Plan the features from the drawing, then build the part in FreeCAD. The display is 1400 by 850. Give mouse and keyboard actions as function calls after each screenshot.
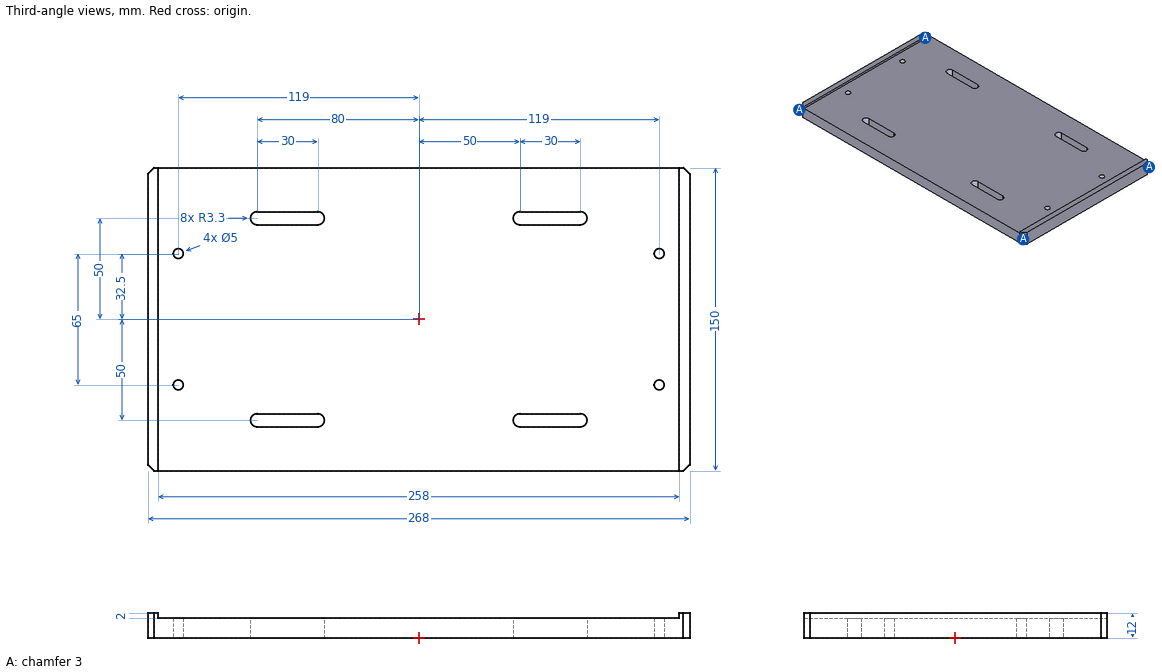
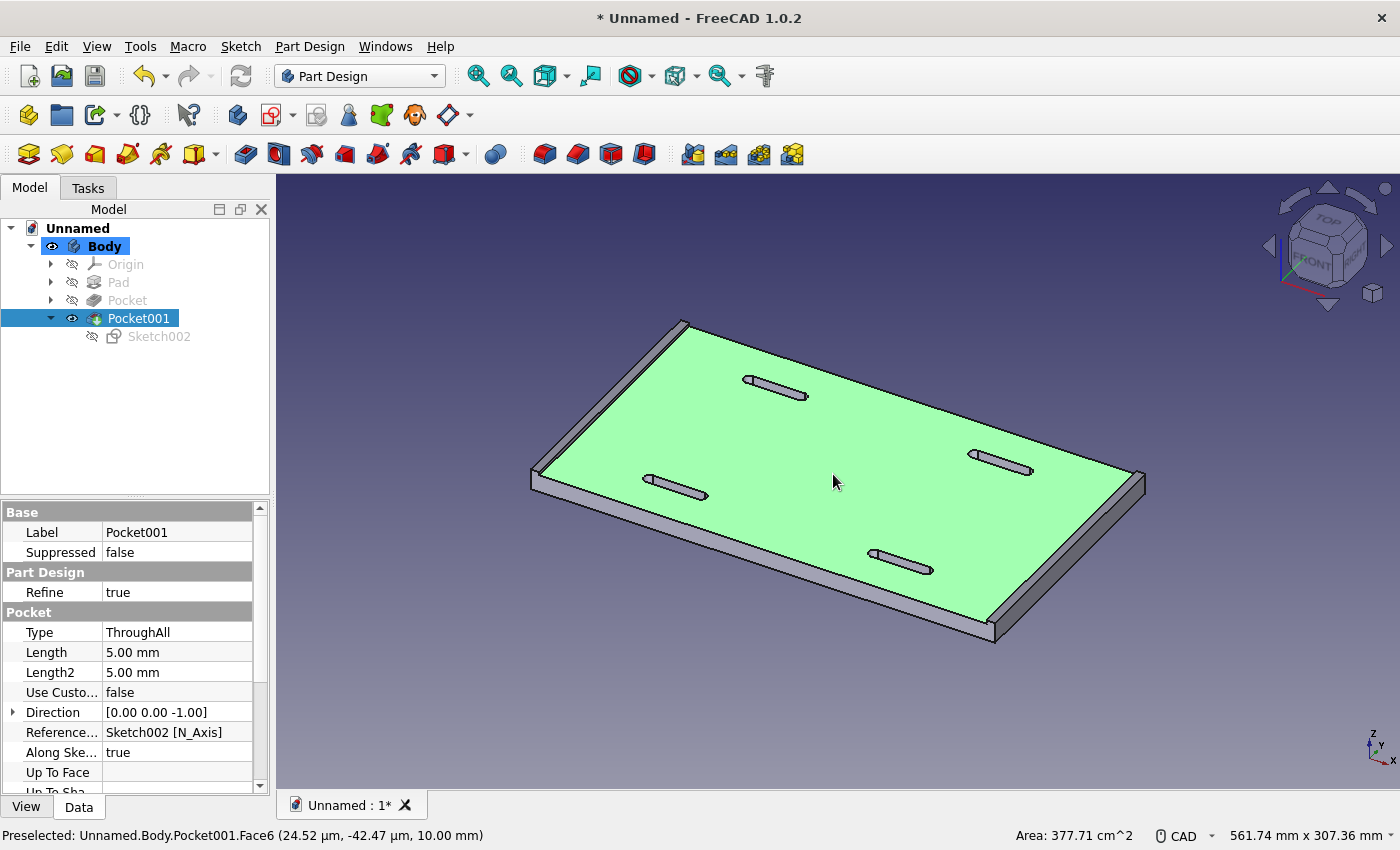
click(270, 116)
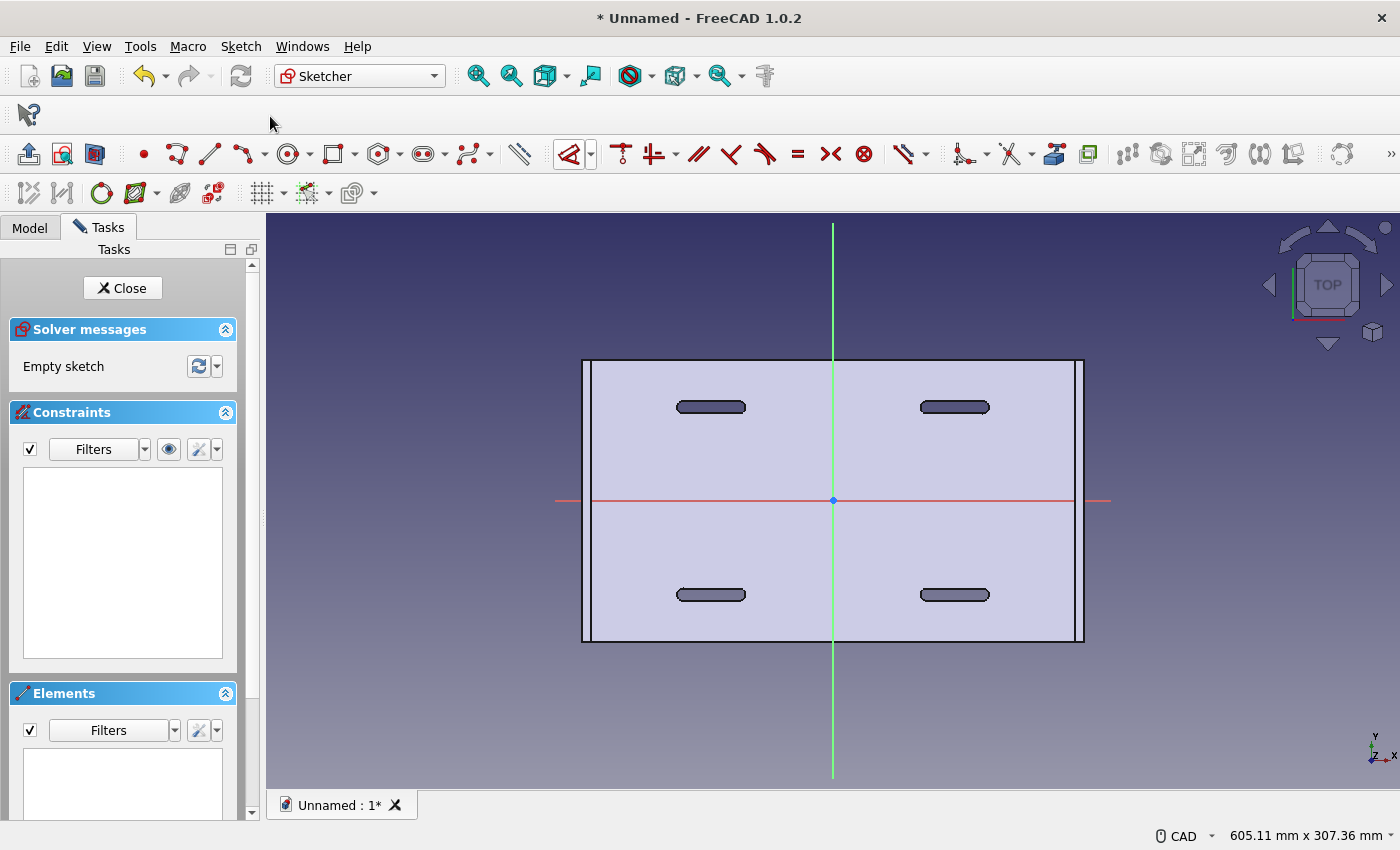
click(95, 154)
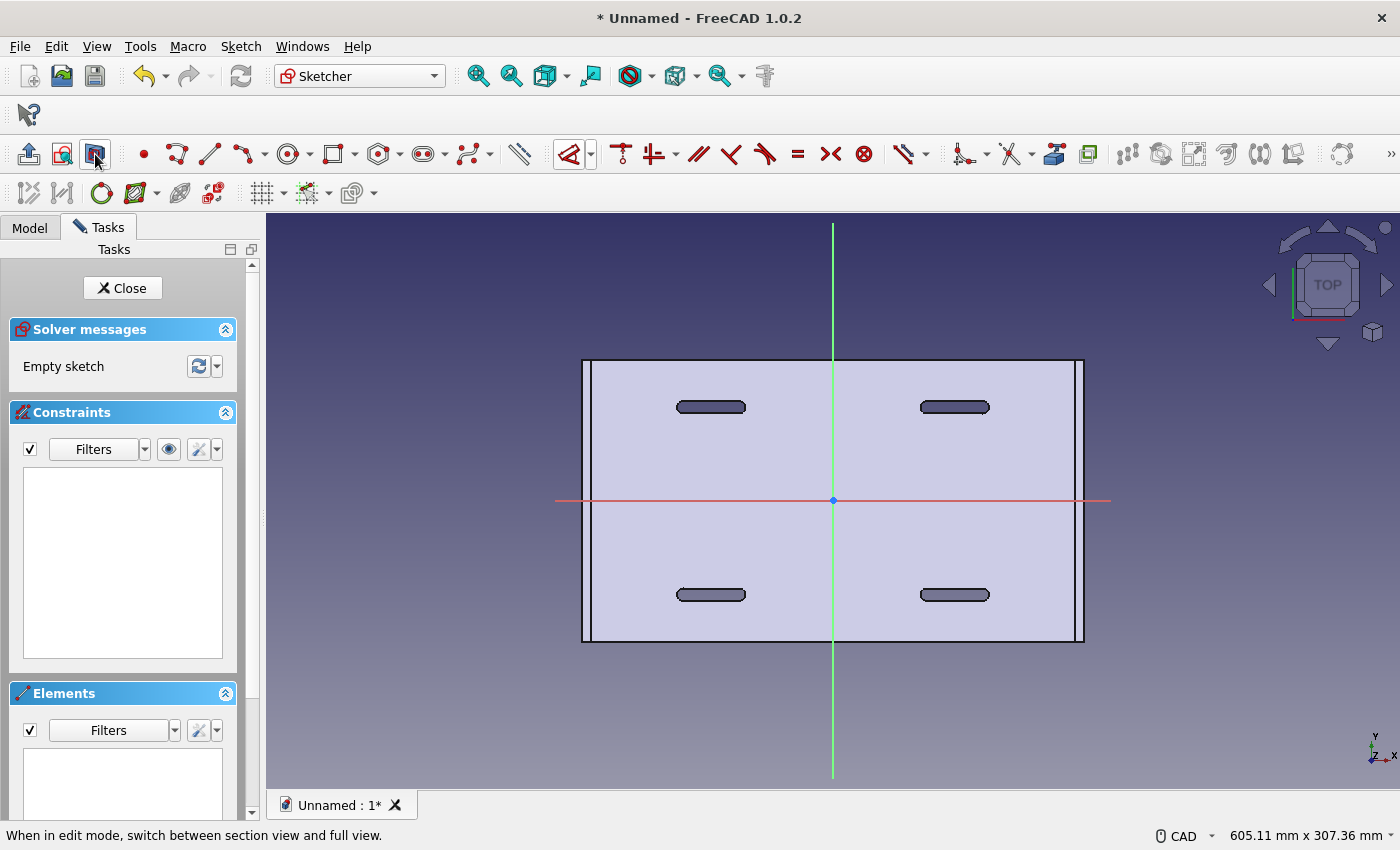
scroll(972, 501, up, 2)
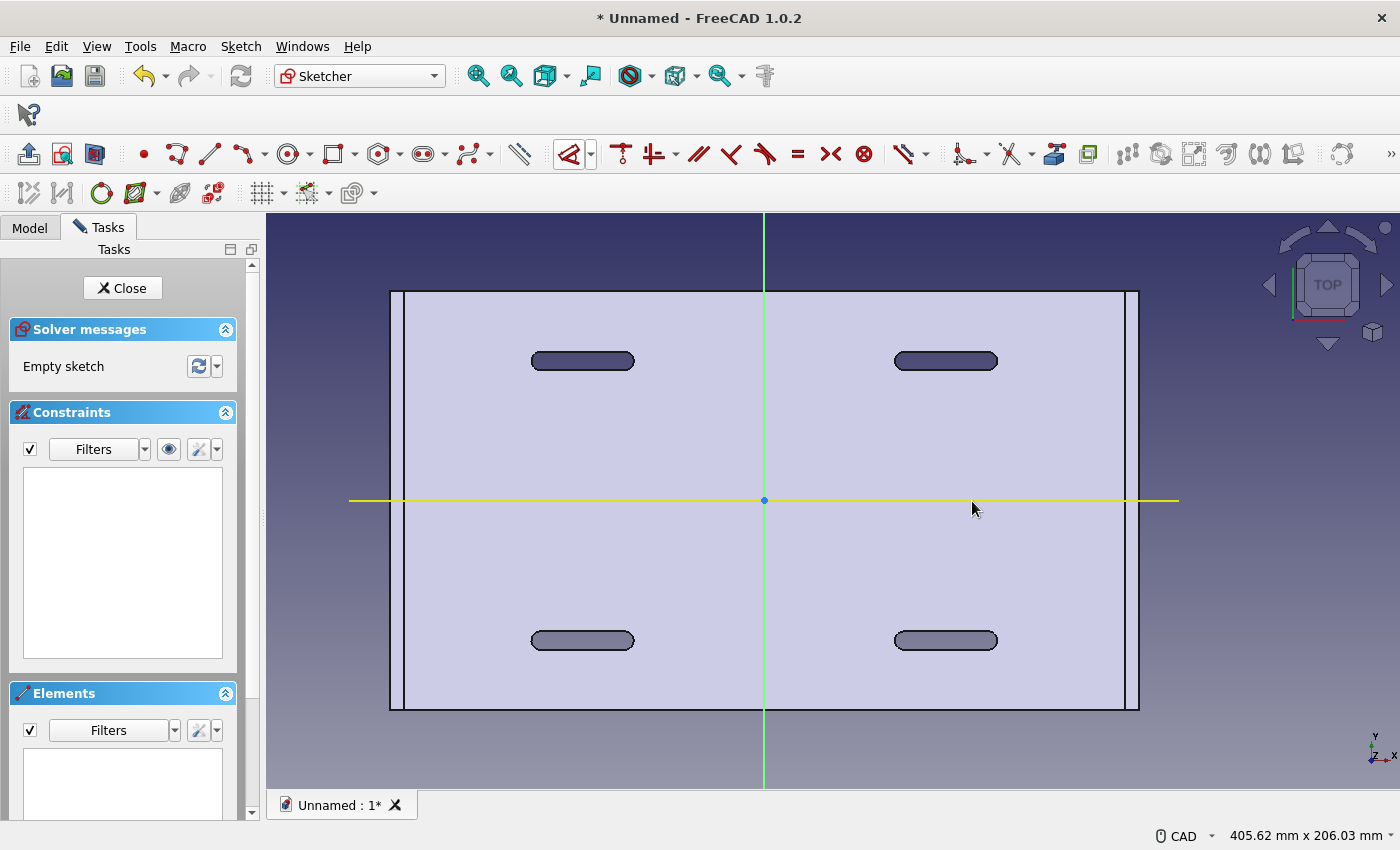
click(288, 154)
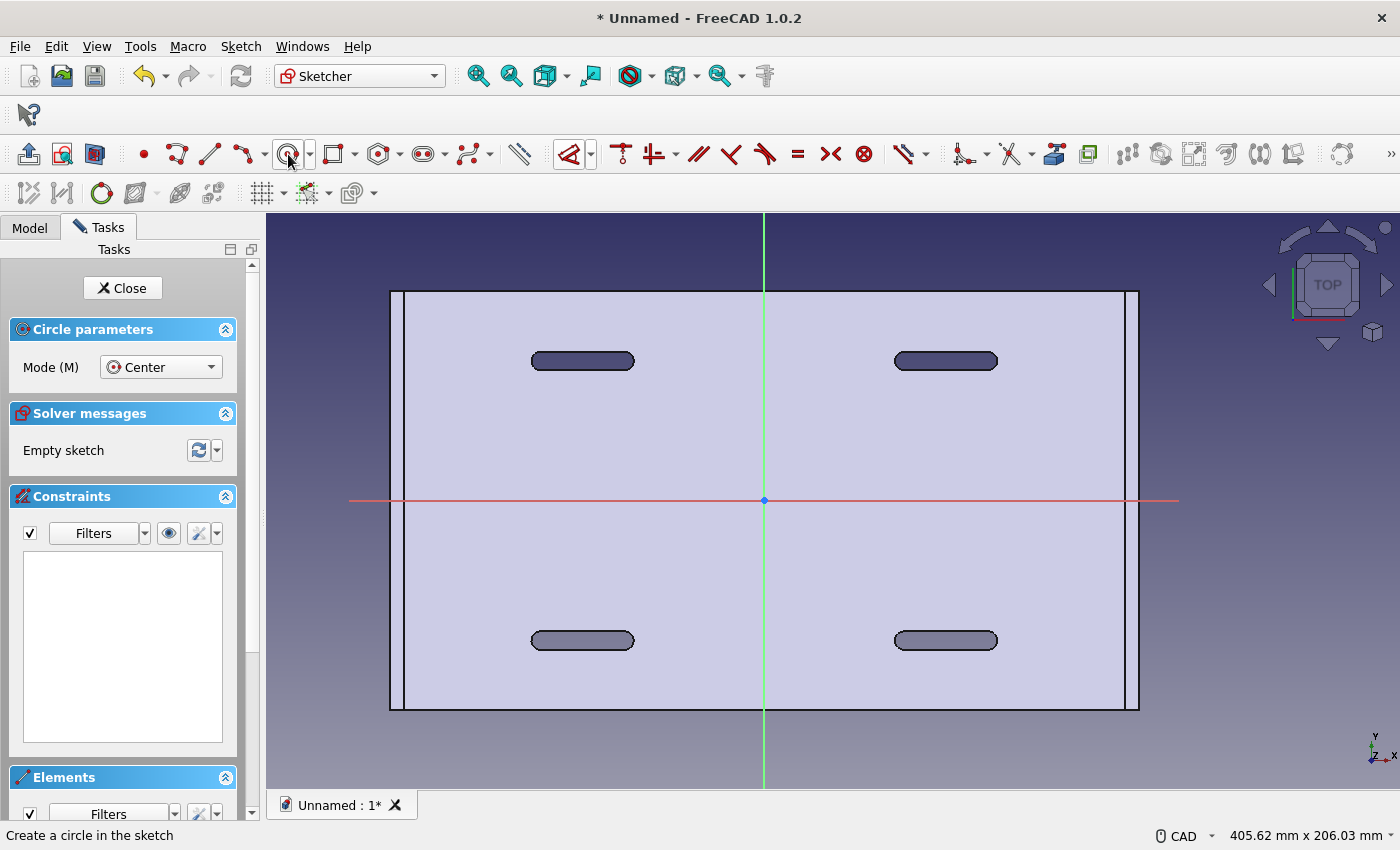
scroll(432, 410, up, 6)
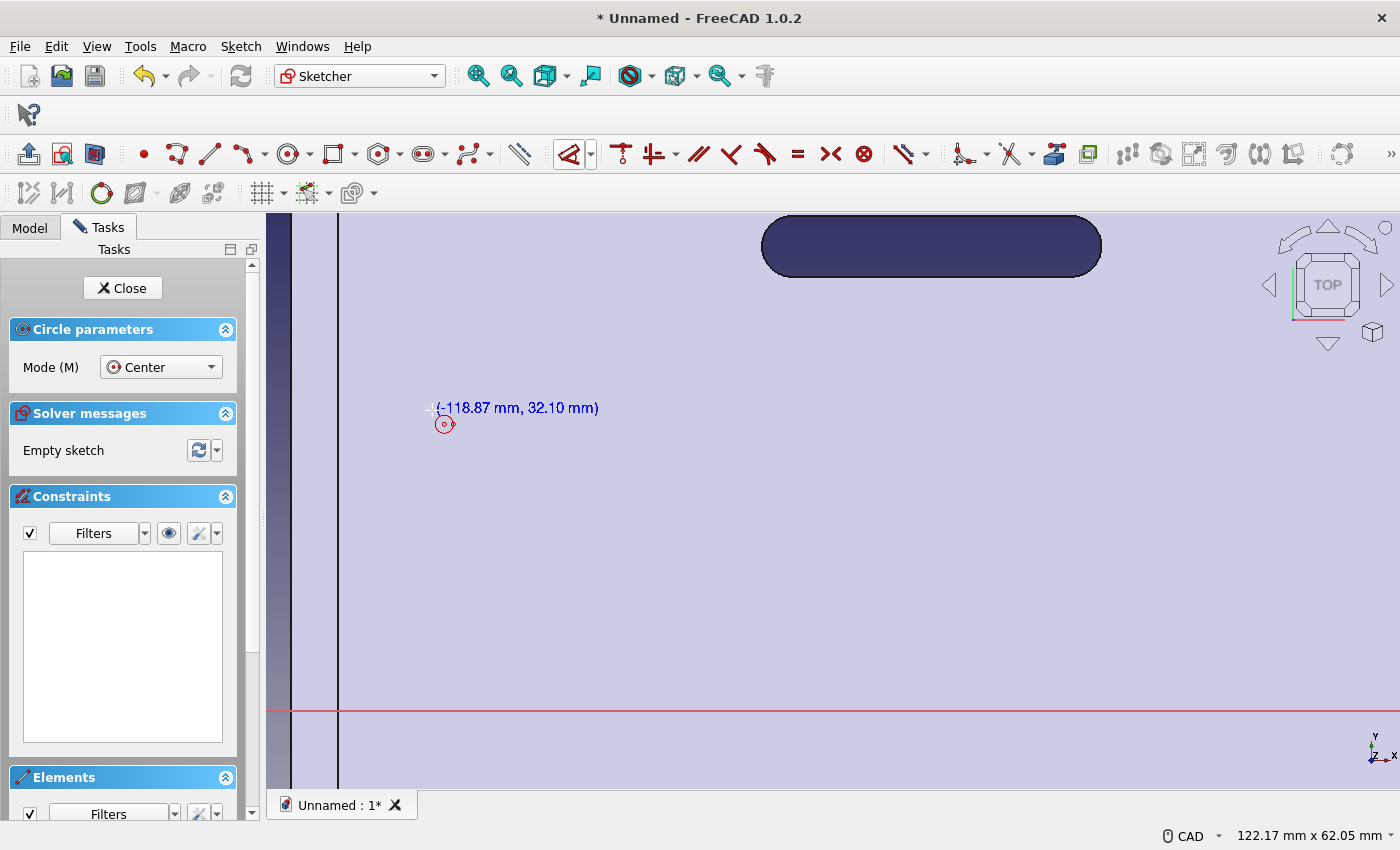
click(430, 409)
move(447, 392)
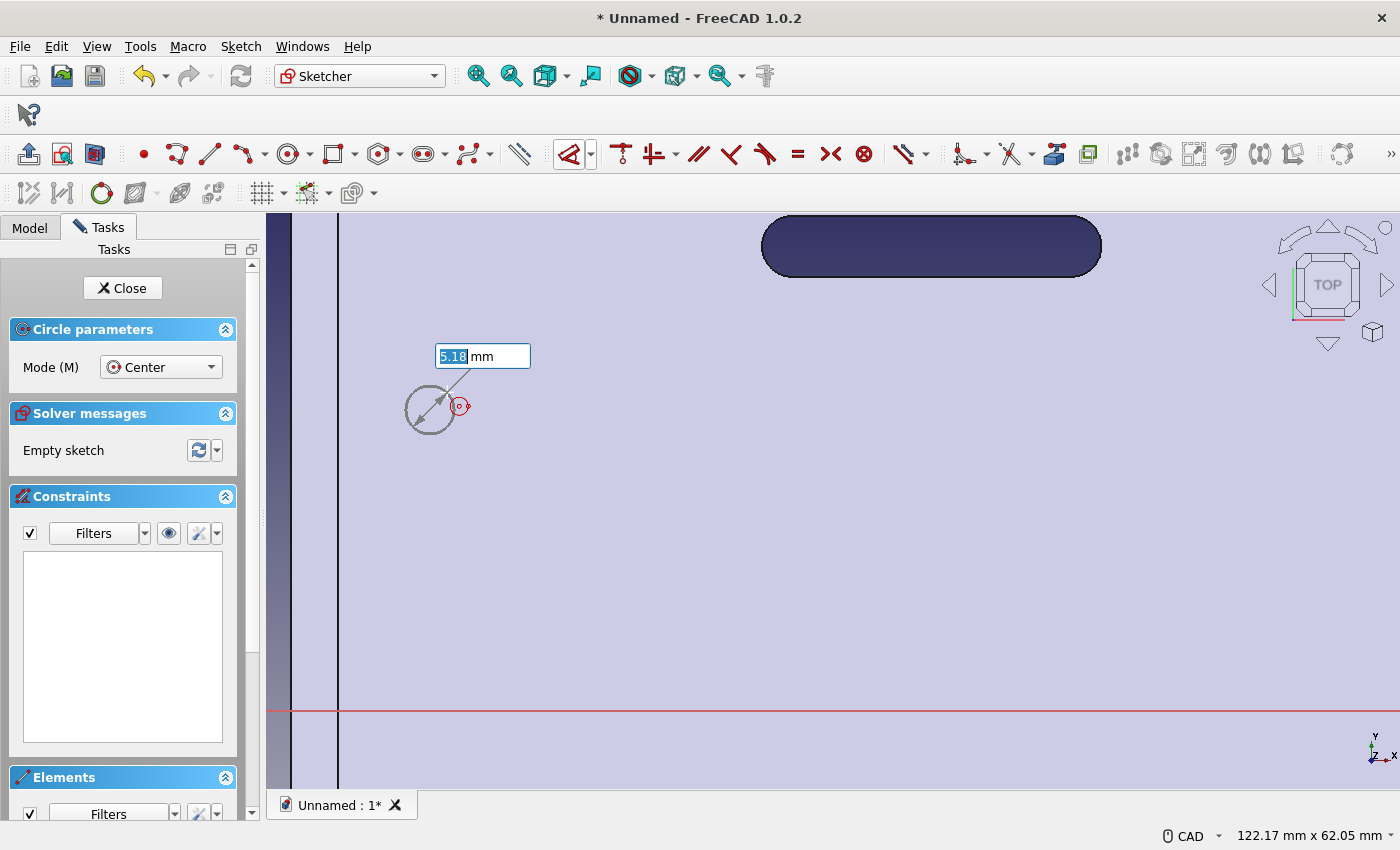
text(5)
key(Return)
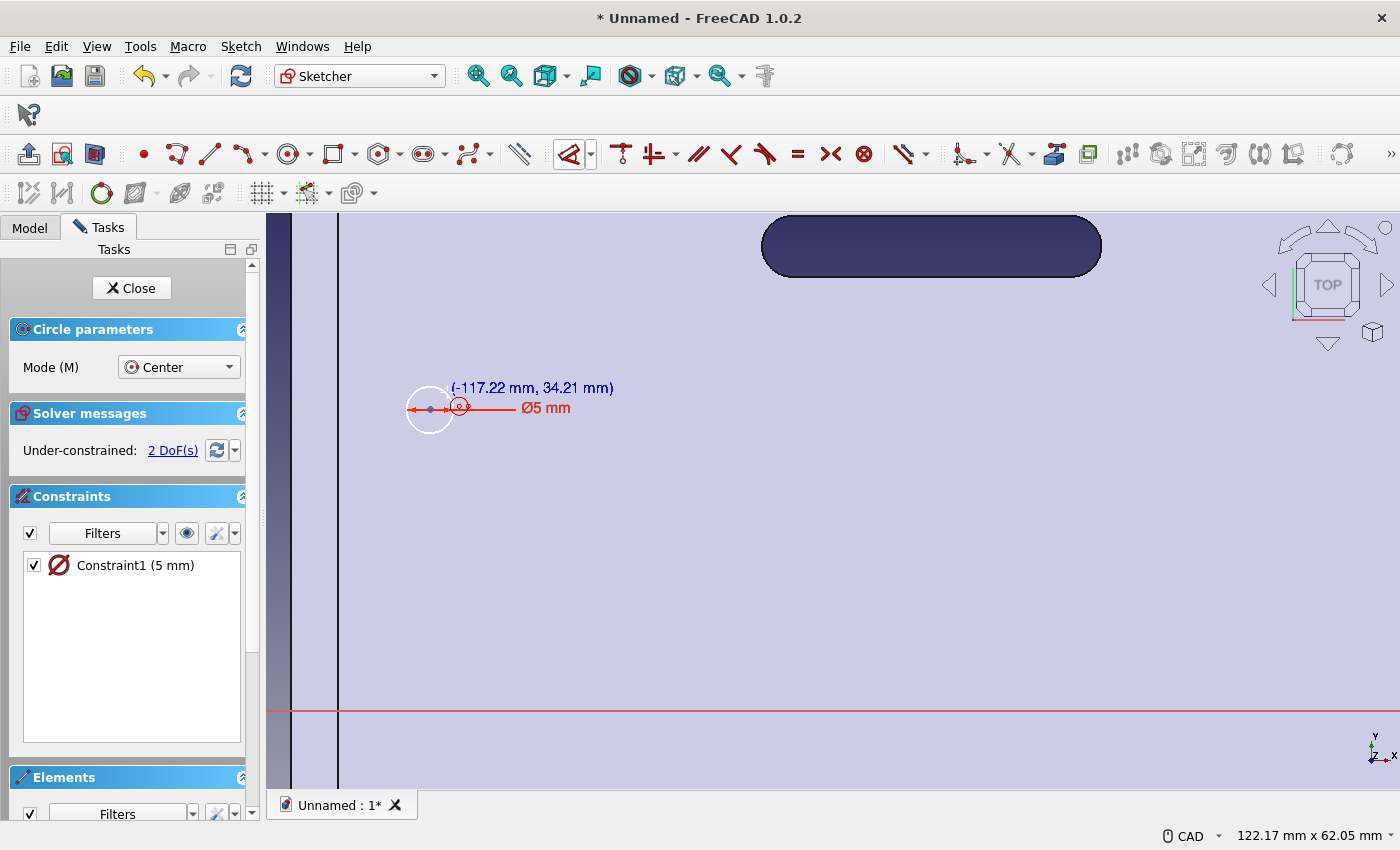
scroll(432, 411, down, 6)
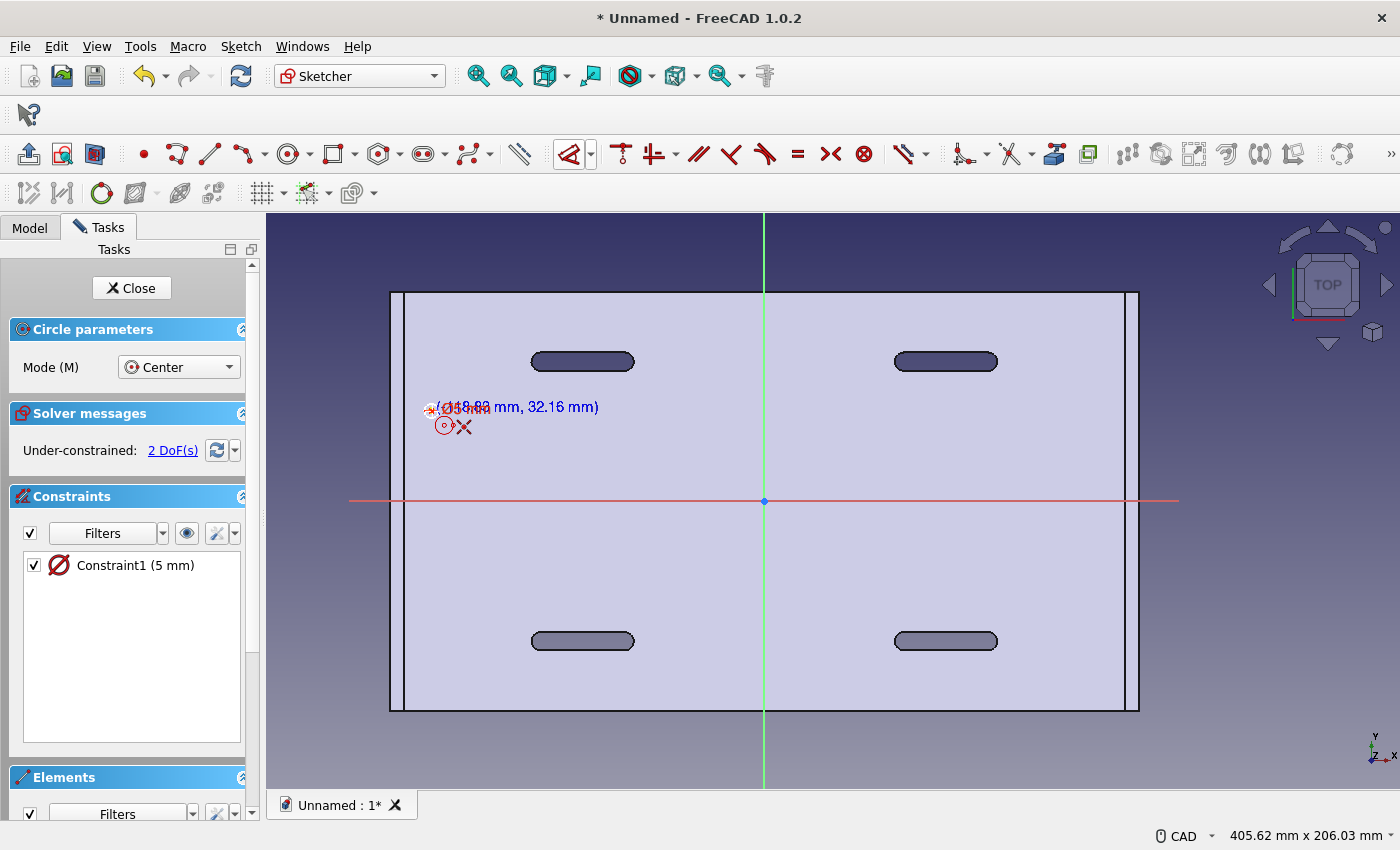
scroll(432, 592, up, 6)